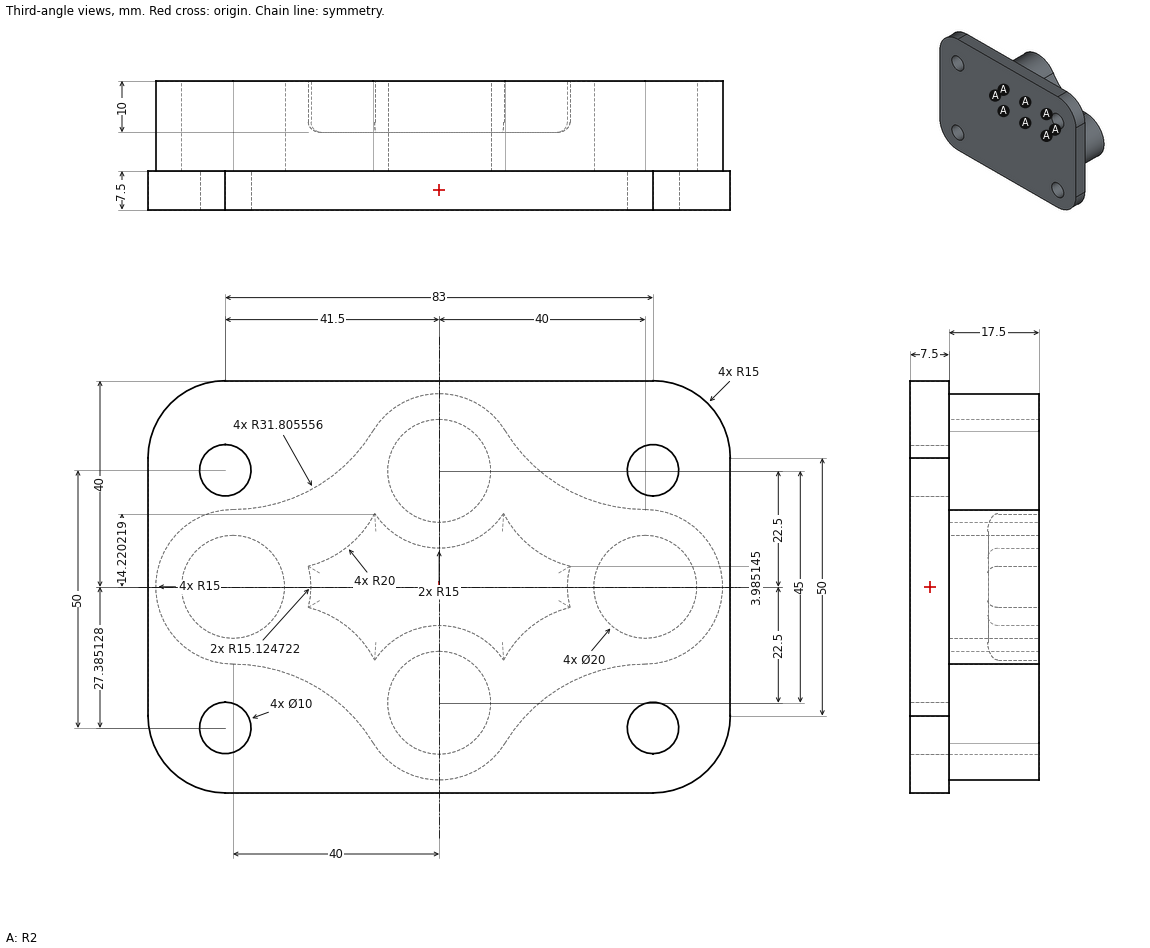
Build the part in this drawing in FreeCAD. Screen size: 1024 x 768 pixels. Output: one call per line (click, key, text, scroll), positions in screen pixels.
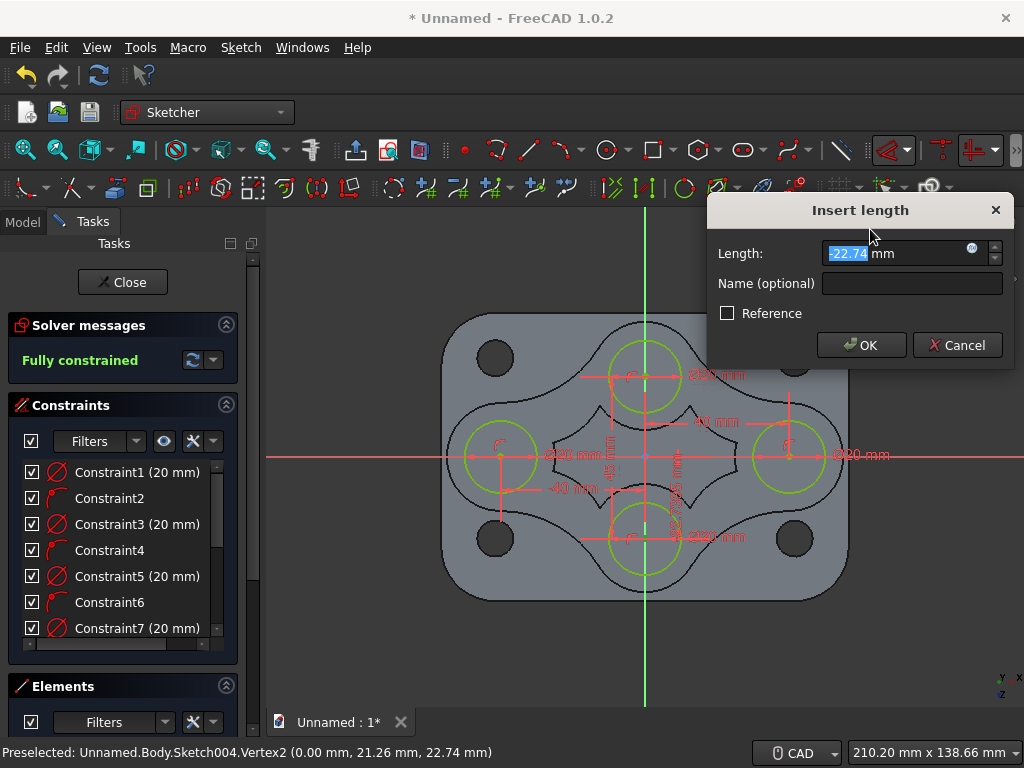
text(-22.5)
key(Return)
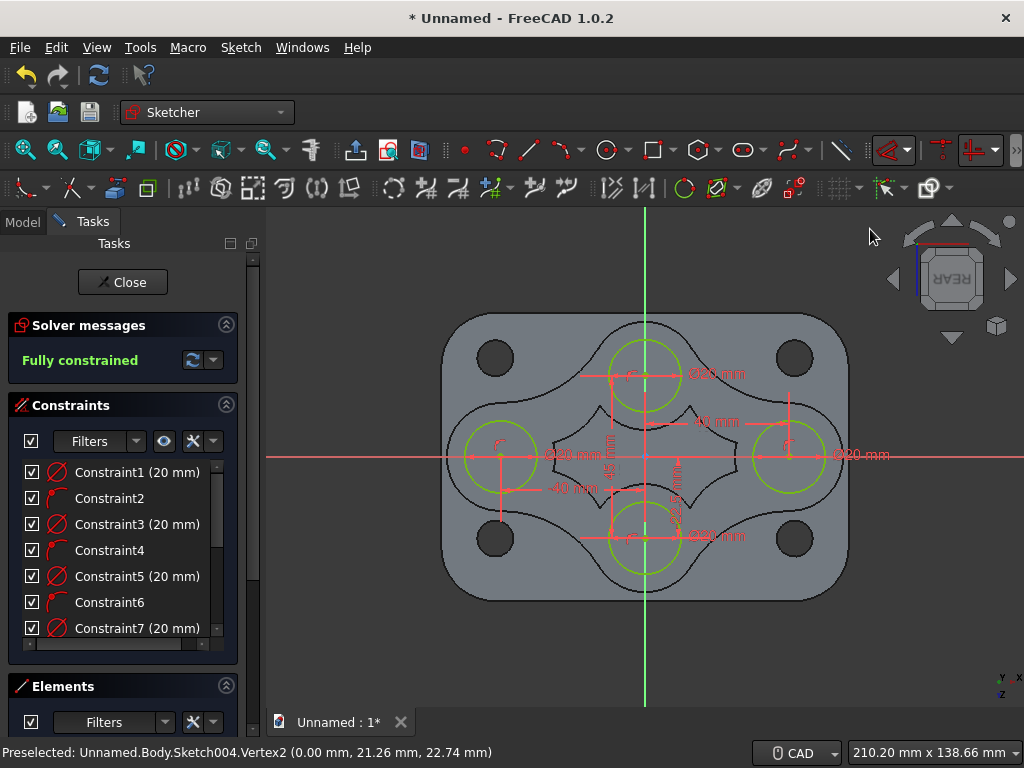
click(123, 282)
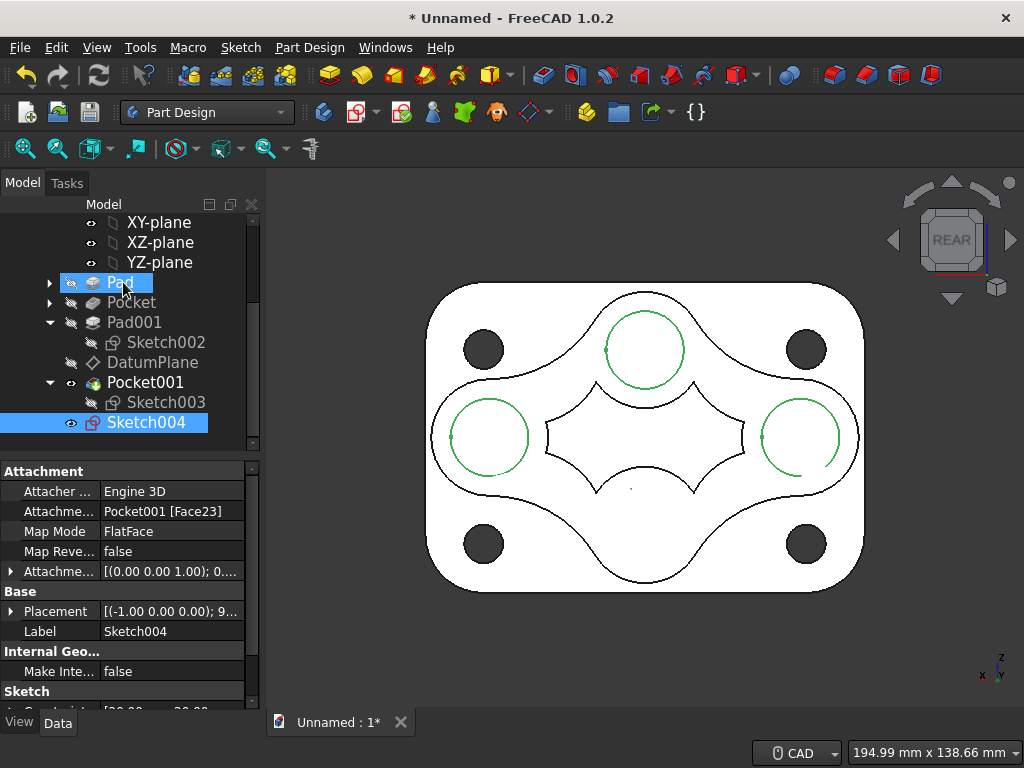
click(544, 76)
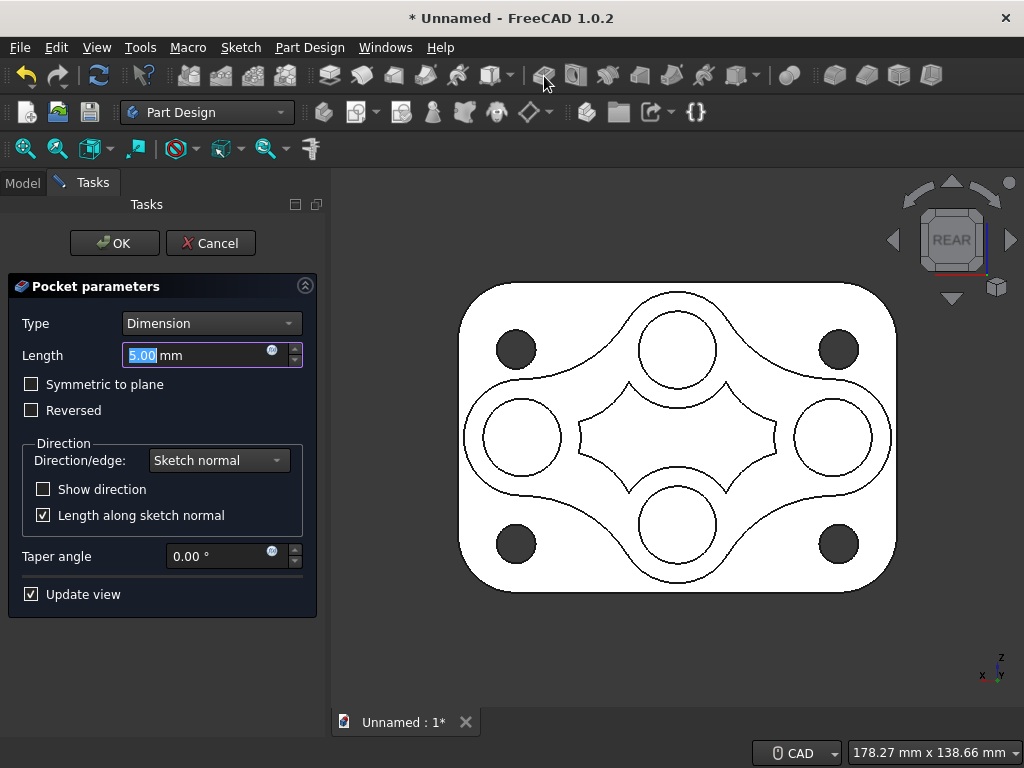
text(17.5)
key(Tab)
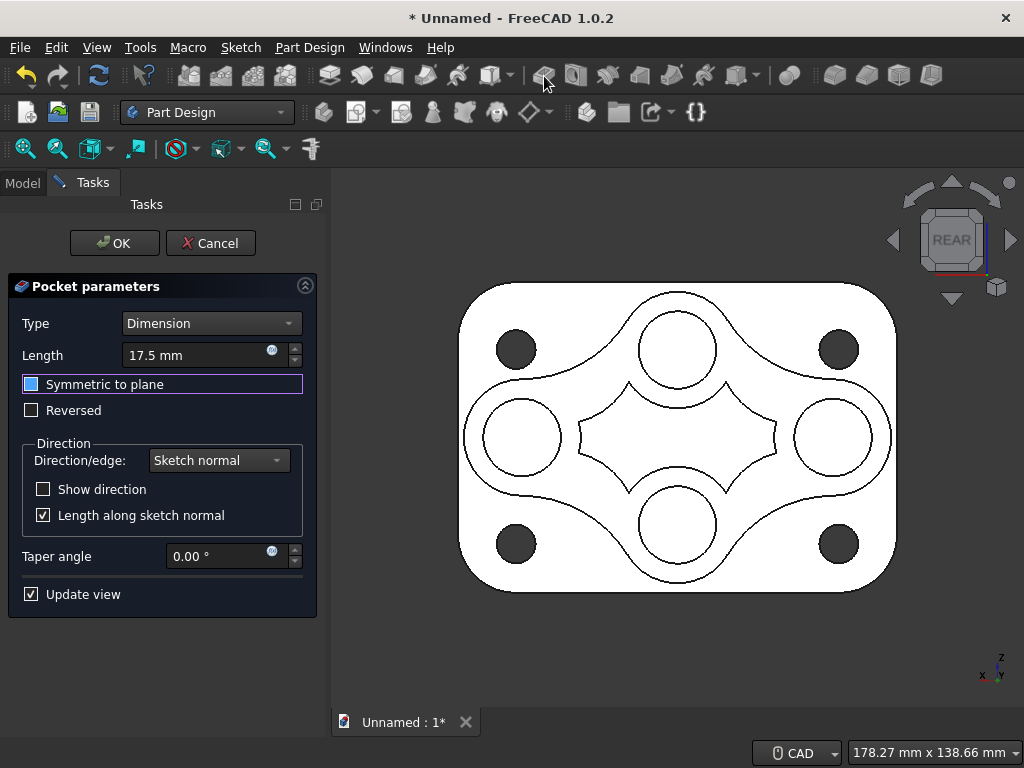
click(115, 243)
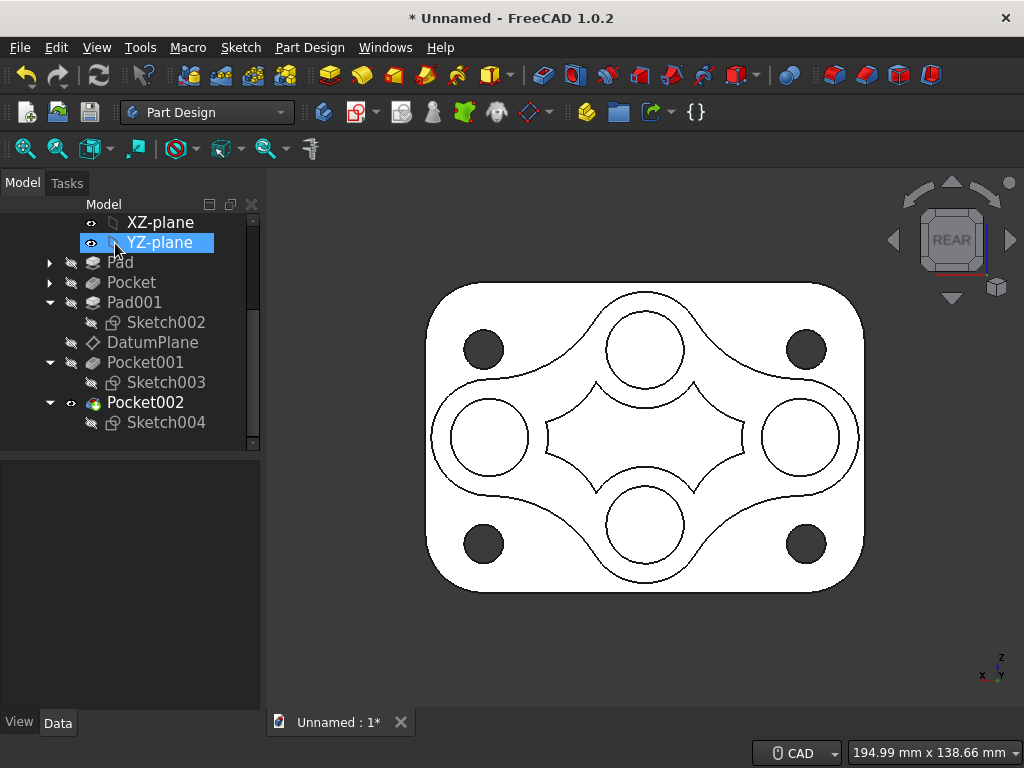
click(673, 436)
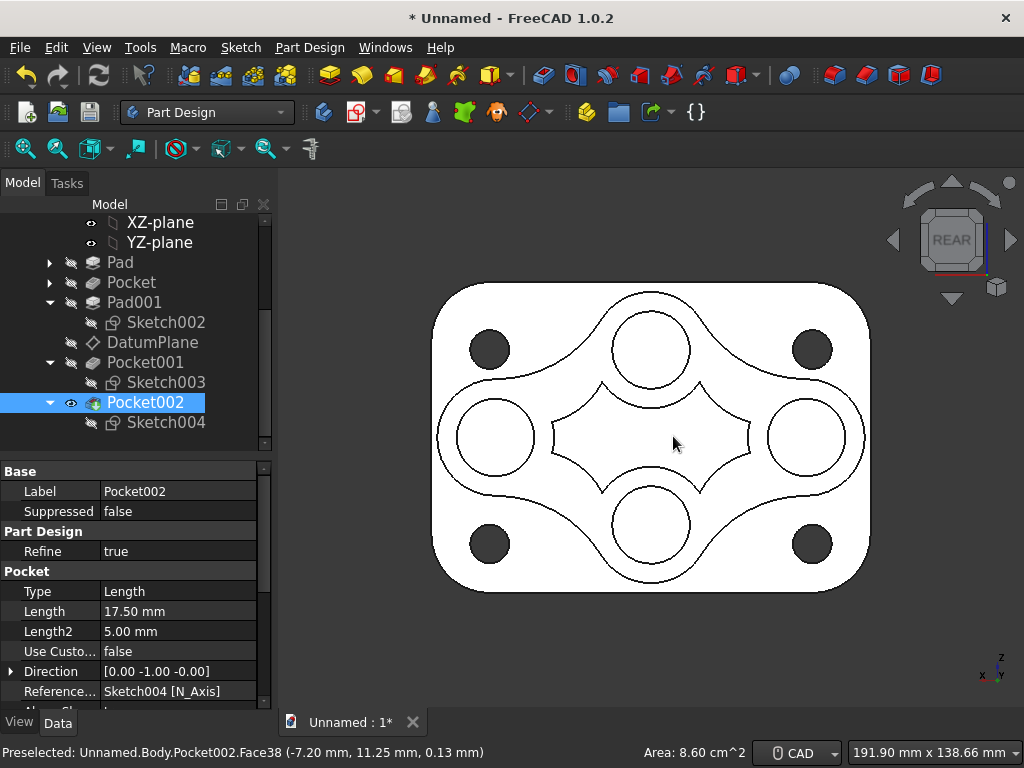
click(836, 76)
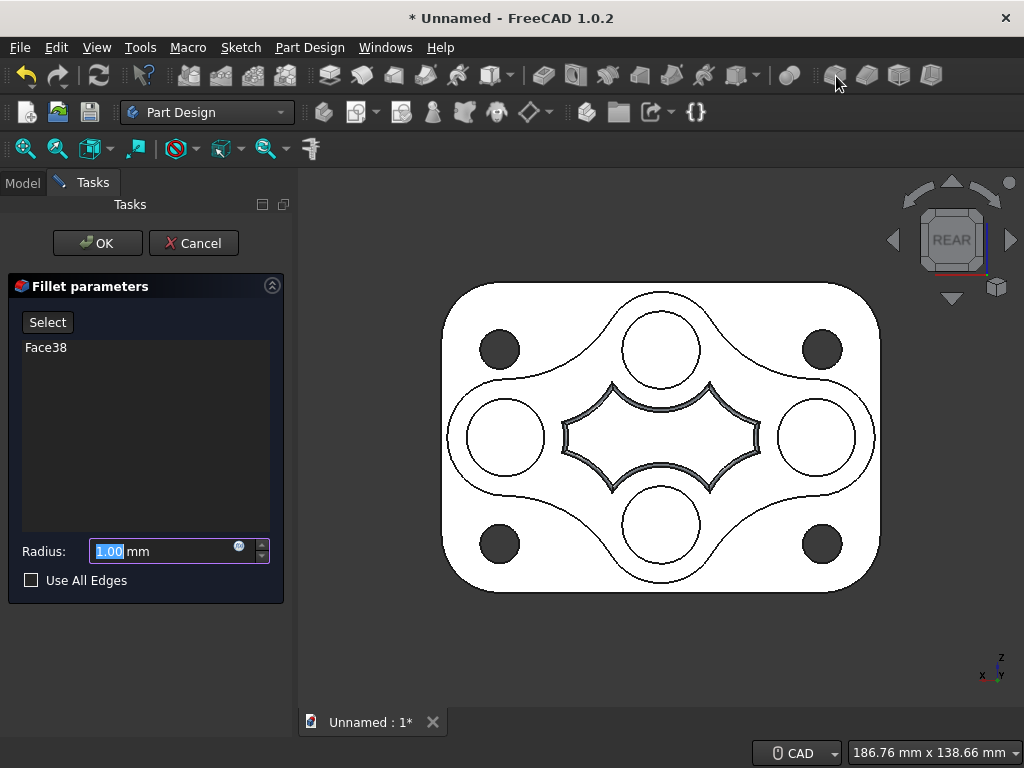
text(2)
key(Tab)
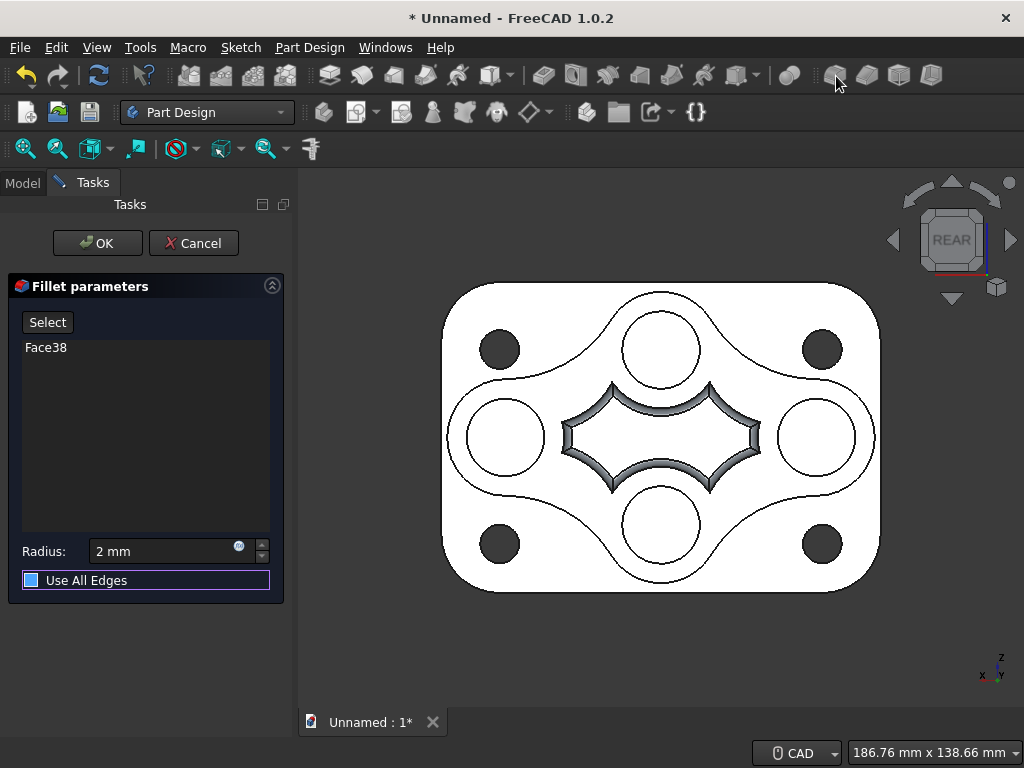
click(98, 243)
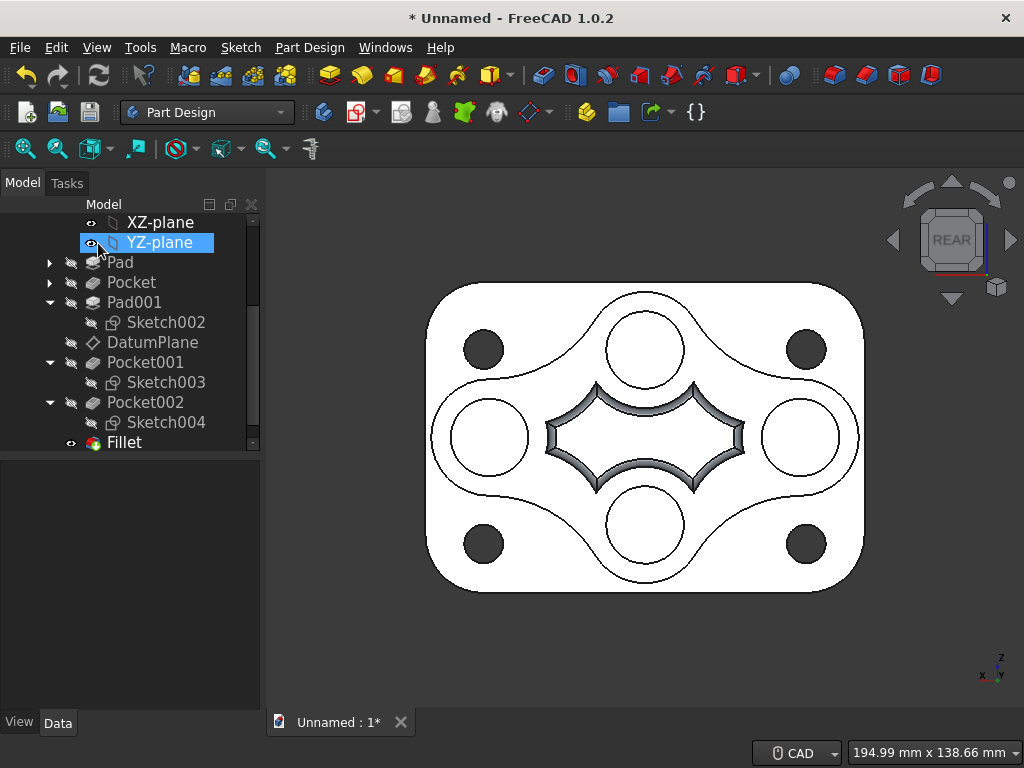
key(0)